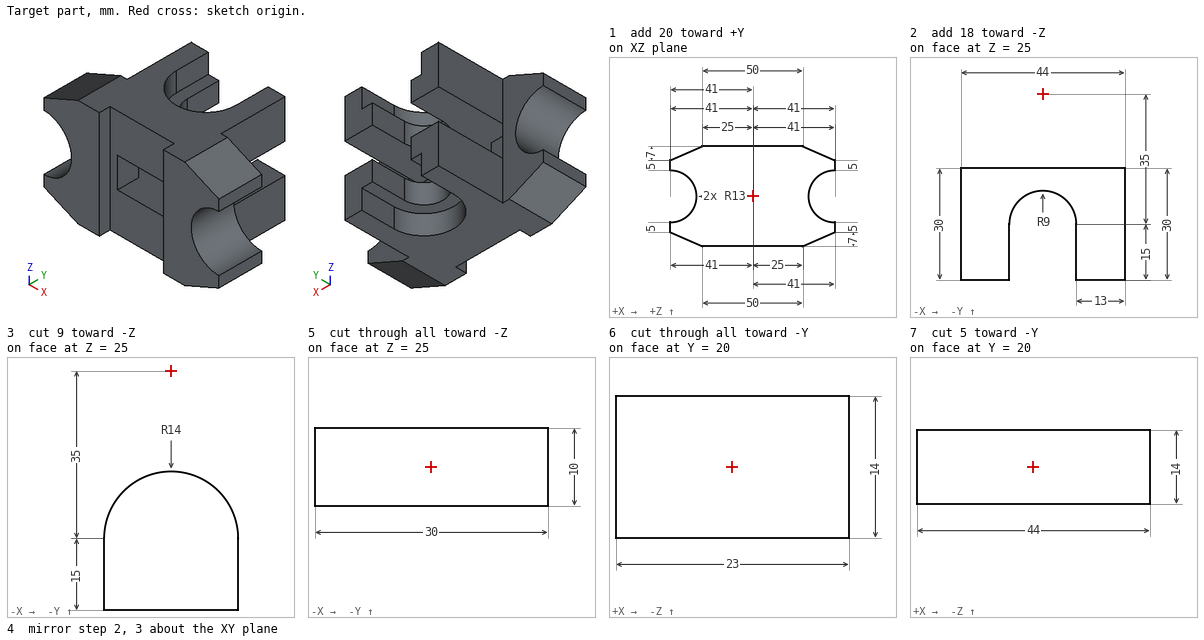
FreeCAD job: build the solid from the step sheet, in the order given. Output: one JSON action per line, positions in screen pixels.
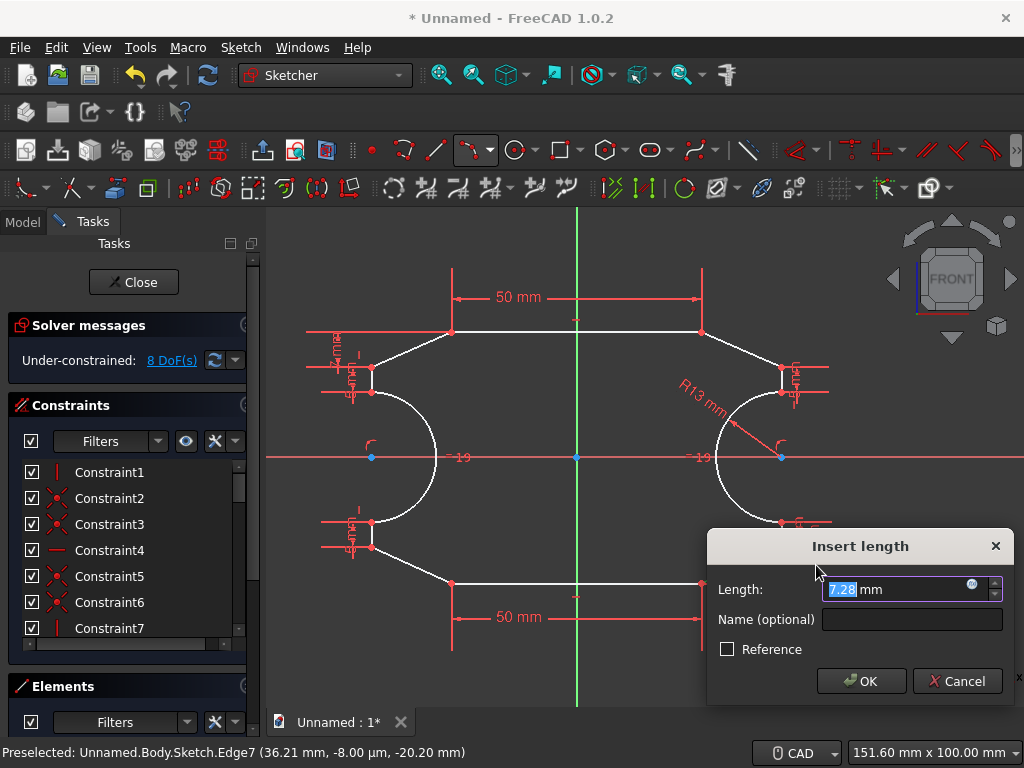
{"action": "type", "text": "7"}
{"action": "key", "text": "Return"}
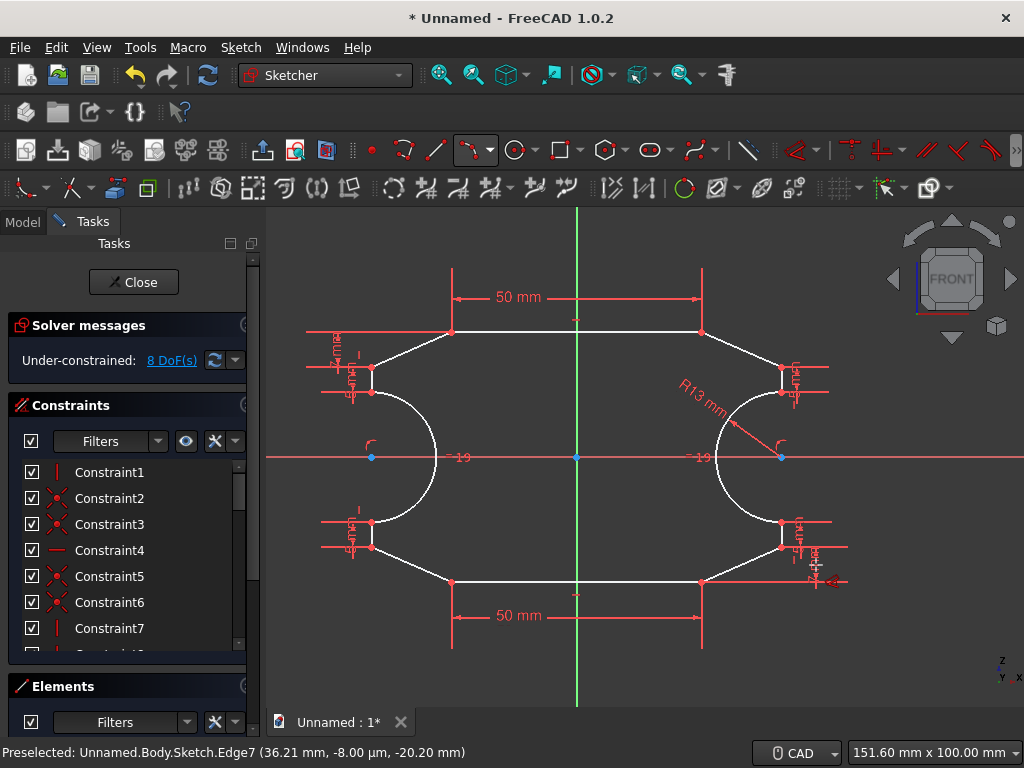
{"action": "left_click", "coordinate": [372, 392]}
{"action": "left_click", "coordinate": [474, 358]}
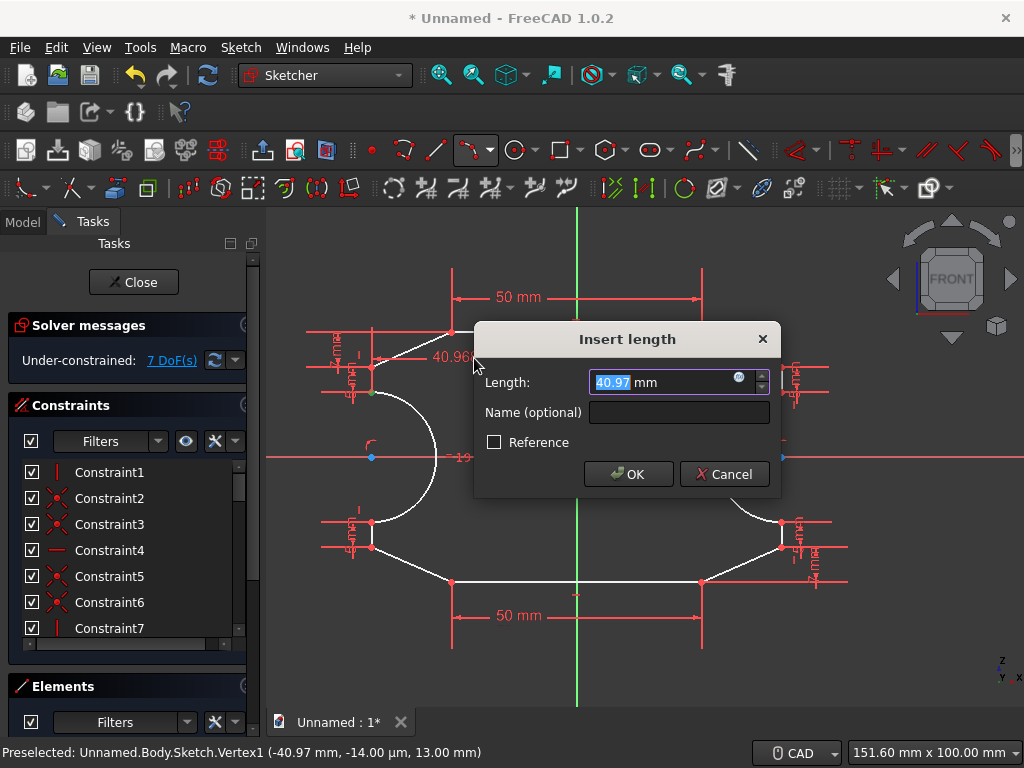
{"action": "type", "text": "41"}
{"action": "key", "text": "Return"}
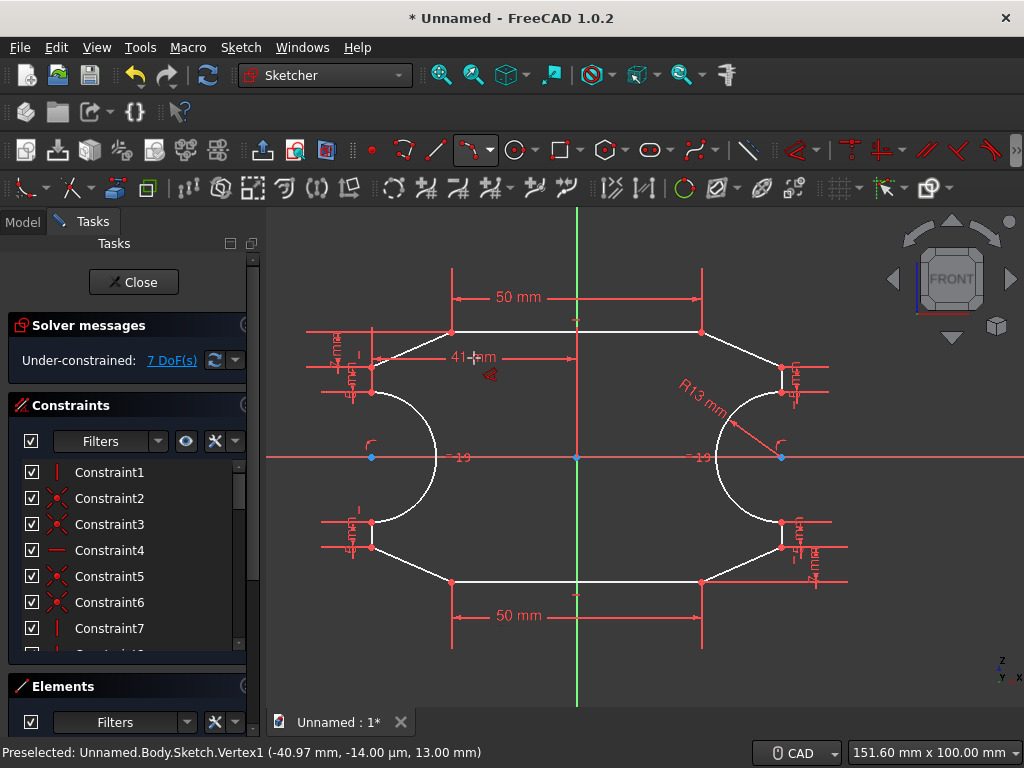
{"action": "left_click", "coordinate": [452, 332]}
{"action": "left_click", "coordinate": [514, 491]}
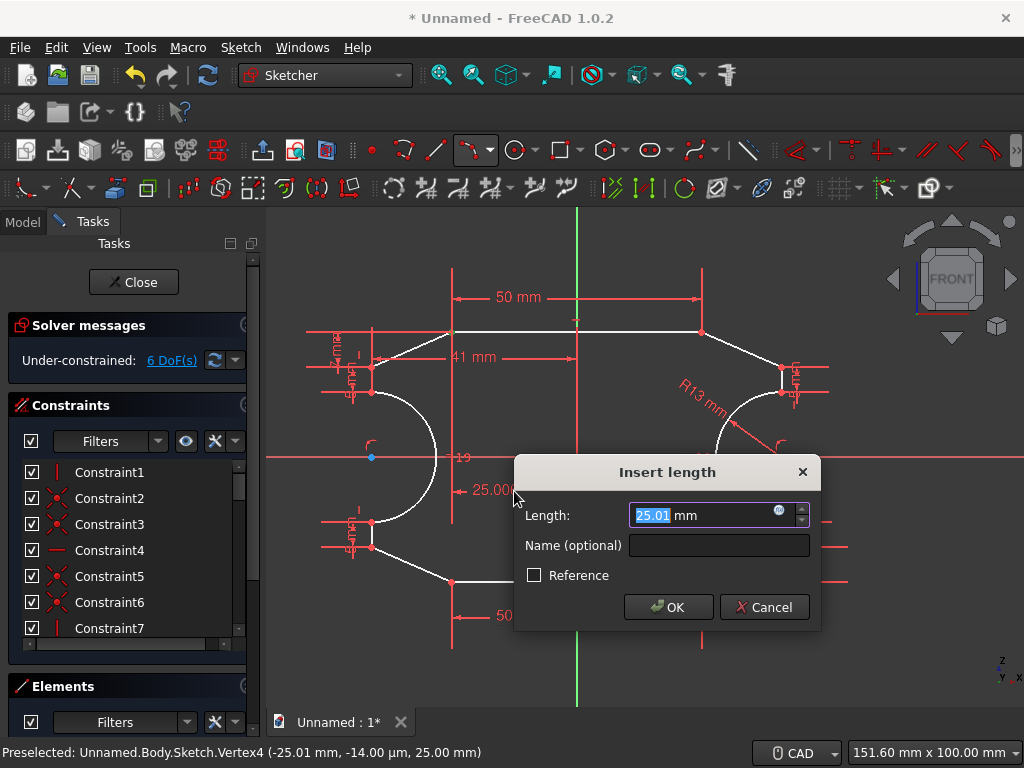
{"action": "type", "text": "25"}
{"action": "key", "text": "Return"}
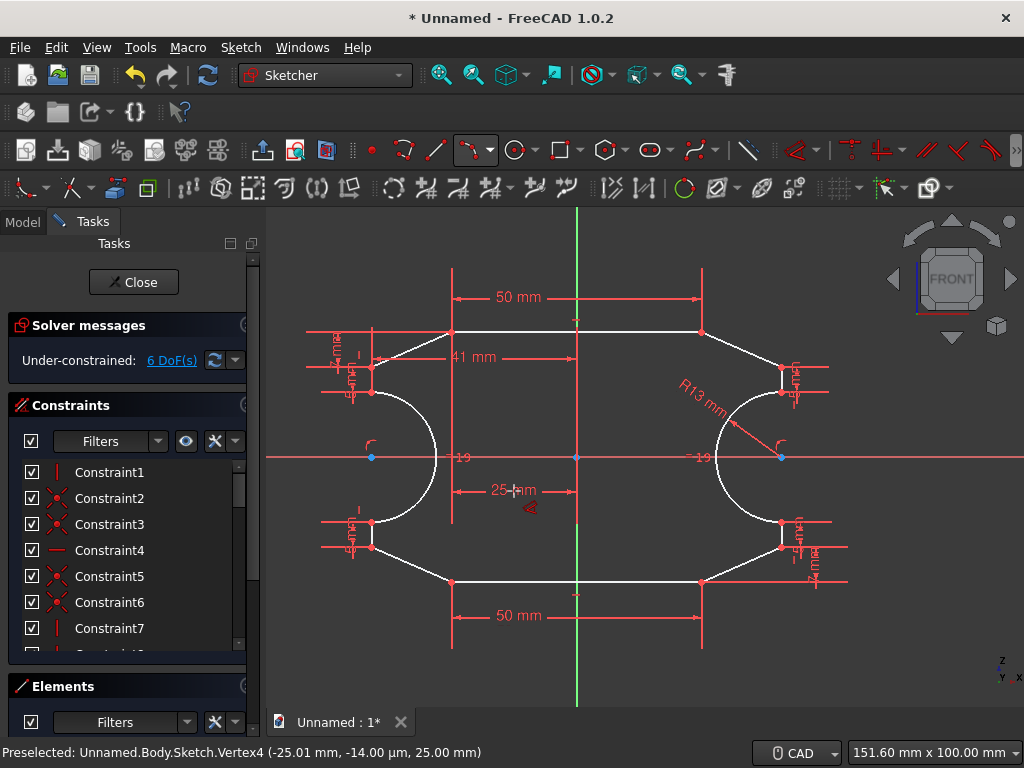
{"action": "left_click", "coordinate": [782, 367]}
{"action": "left_click", "coordinate": [751, 333]}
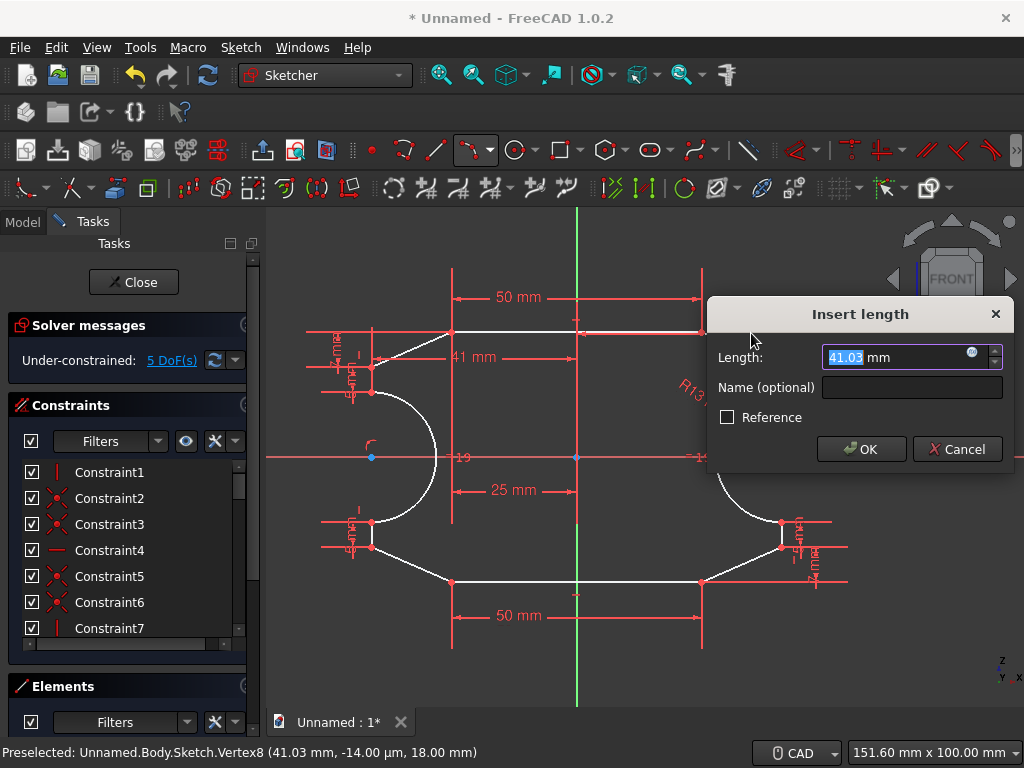
{"action": "type", "text": "41"}
{"action": "key", "text": "Return"}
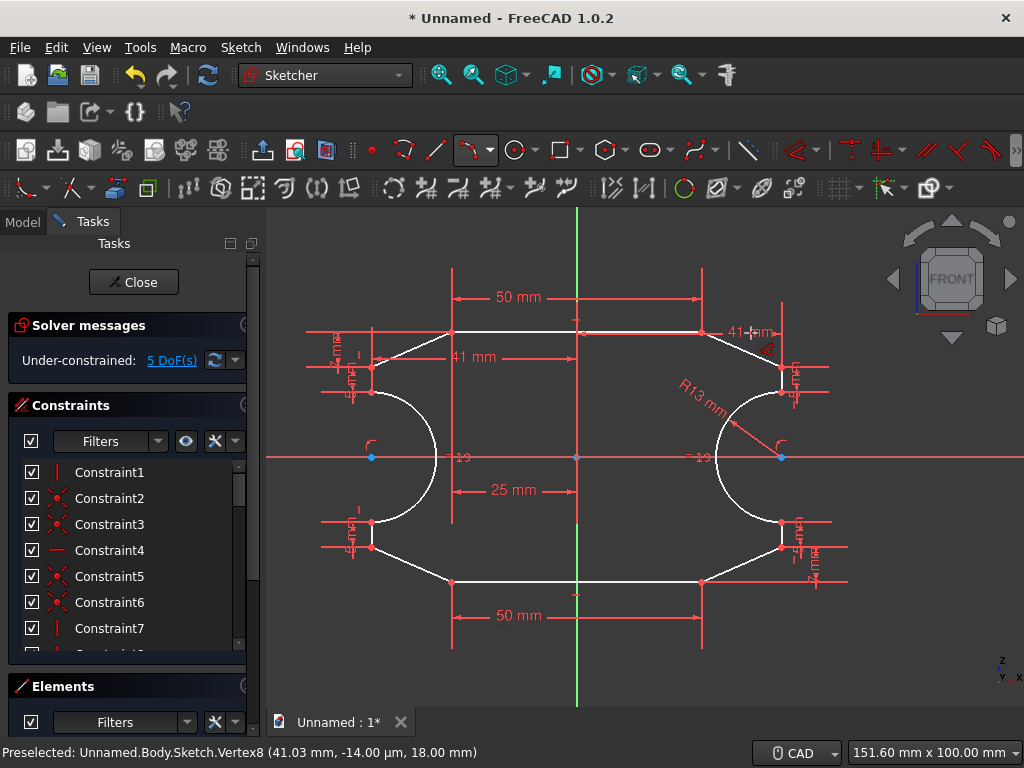
{"action": "left_click", "coordinate": [782, 522]}
{"action": "left_click", "coordinate": [679, 556]}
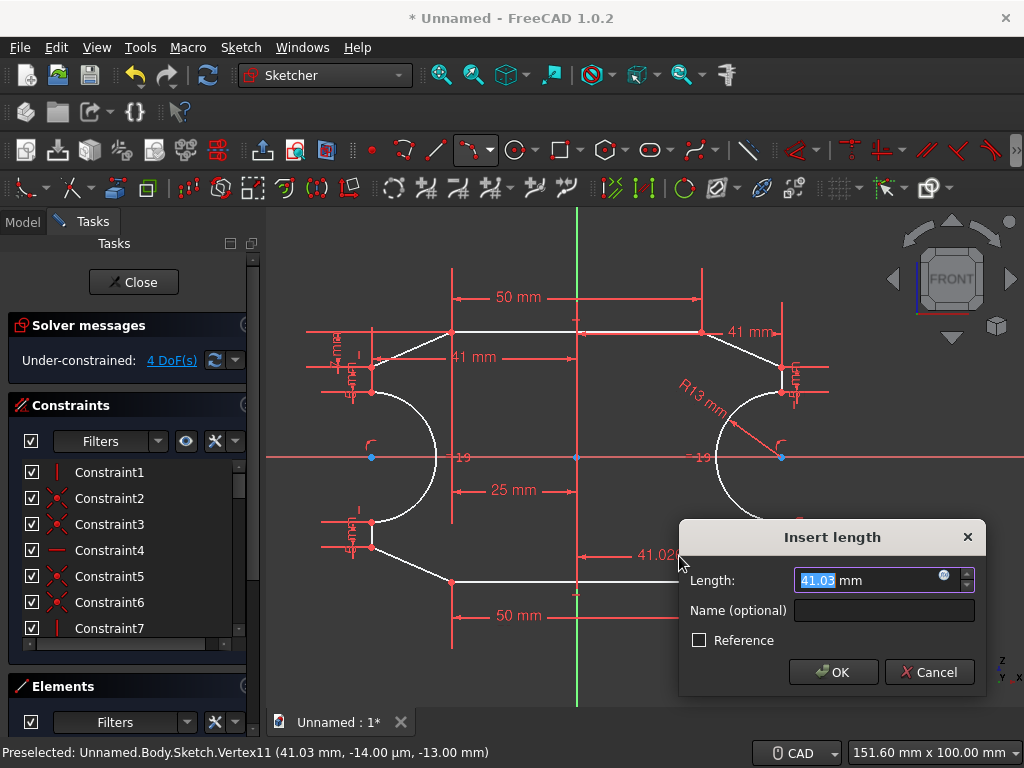
{"action": "type", "text": "41"}
{"action": "key", "text": "Return"}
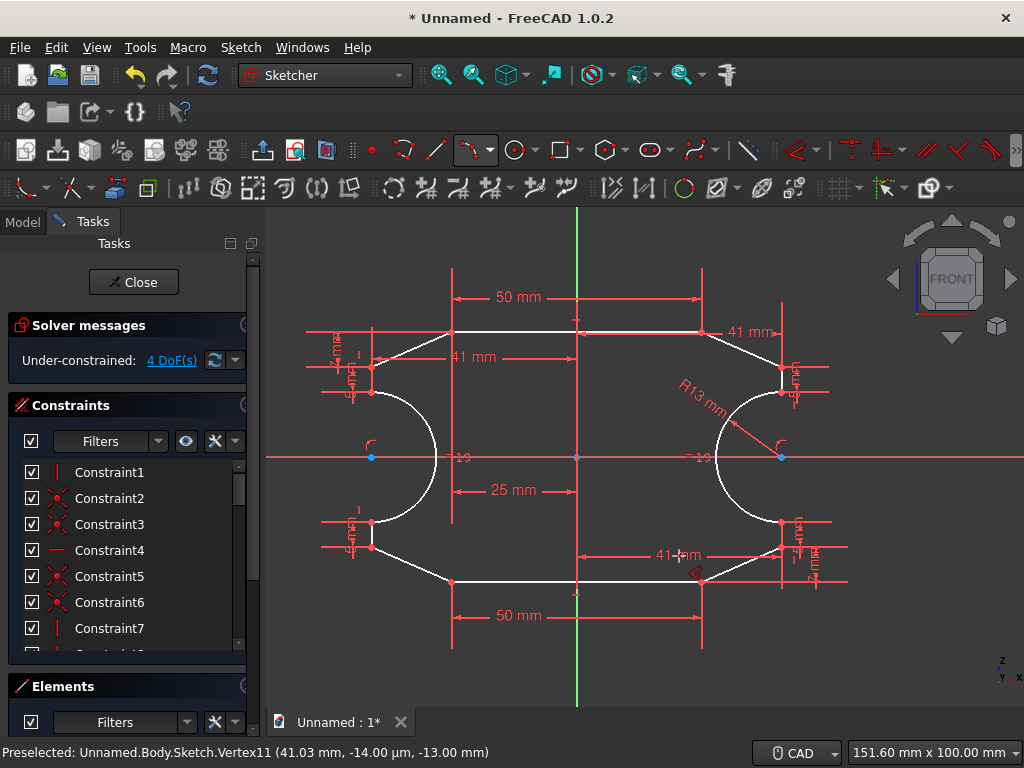
{"action": "left_click", "coordinate": [702, 582]}
{"action": "left_click", "coordinate": [639, 616]}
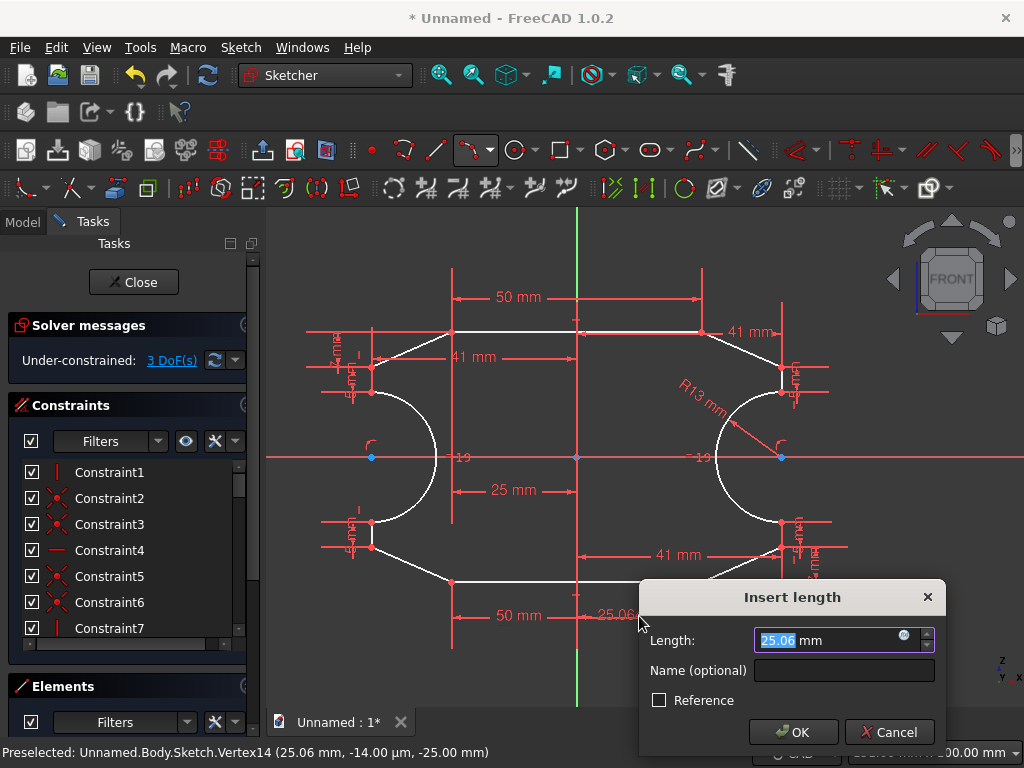
{"action": "type", "text": "25"}
{"action": "key", "text": "Return"}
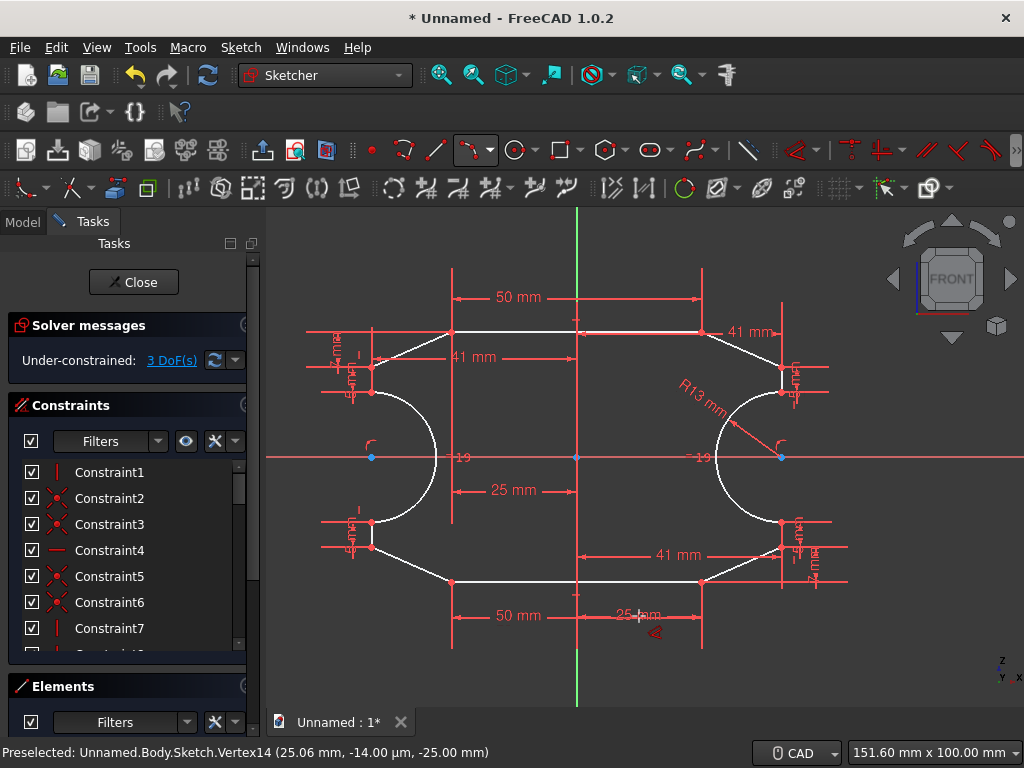
{"action": "left_click", "coordinate": [372, 547]}
{"action": "left_click", "coordinate": [402, 581]}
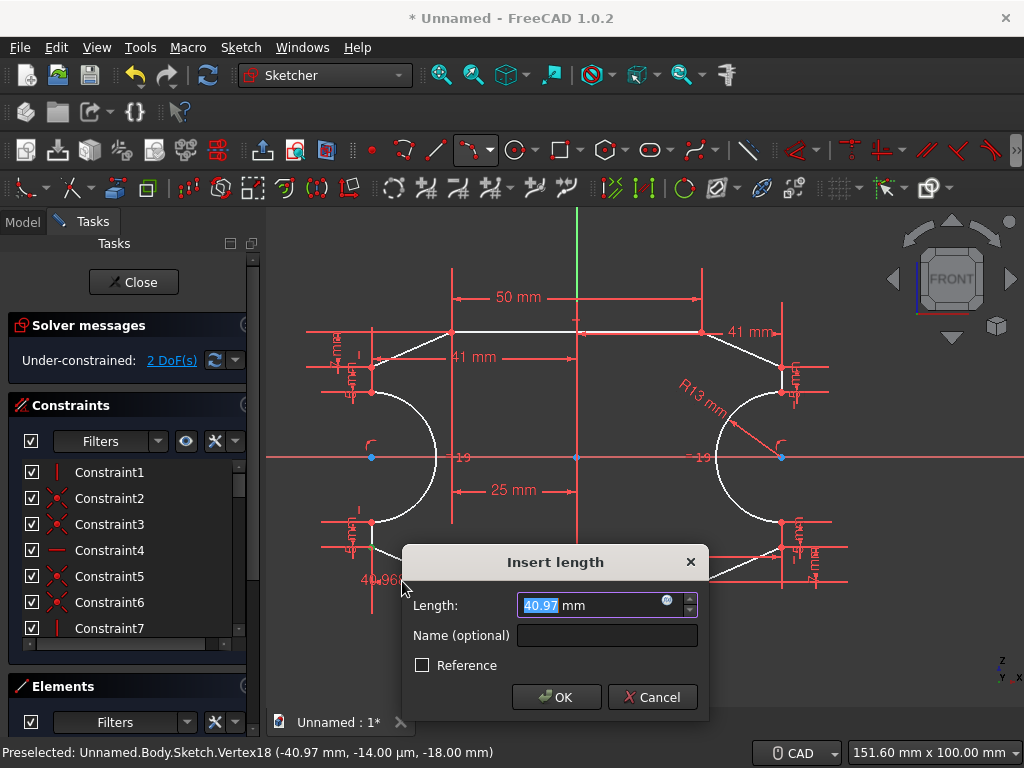
{"action": "type", "text": "41"}
{"action": "key", "text": "Return"}